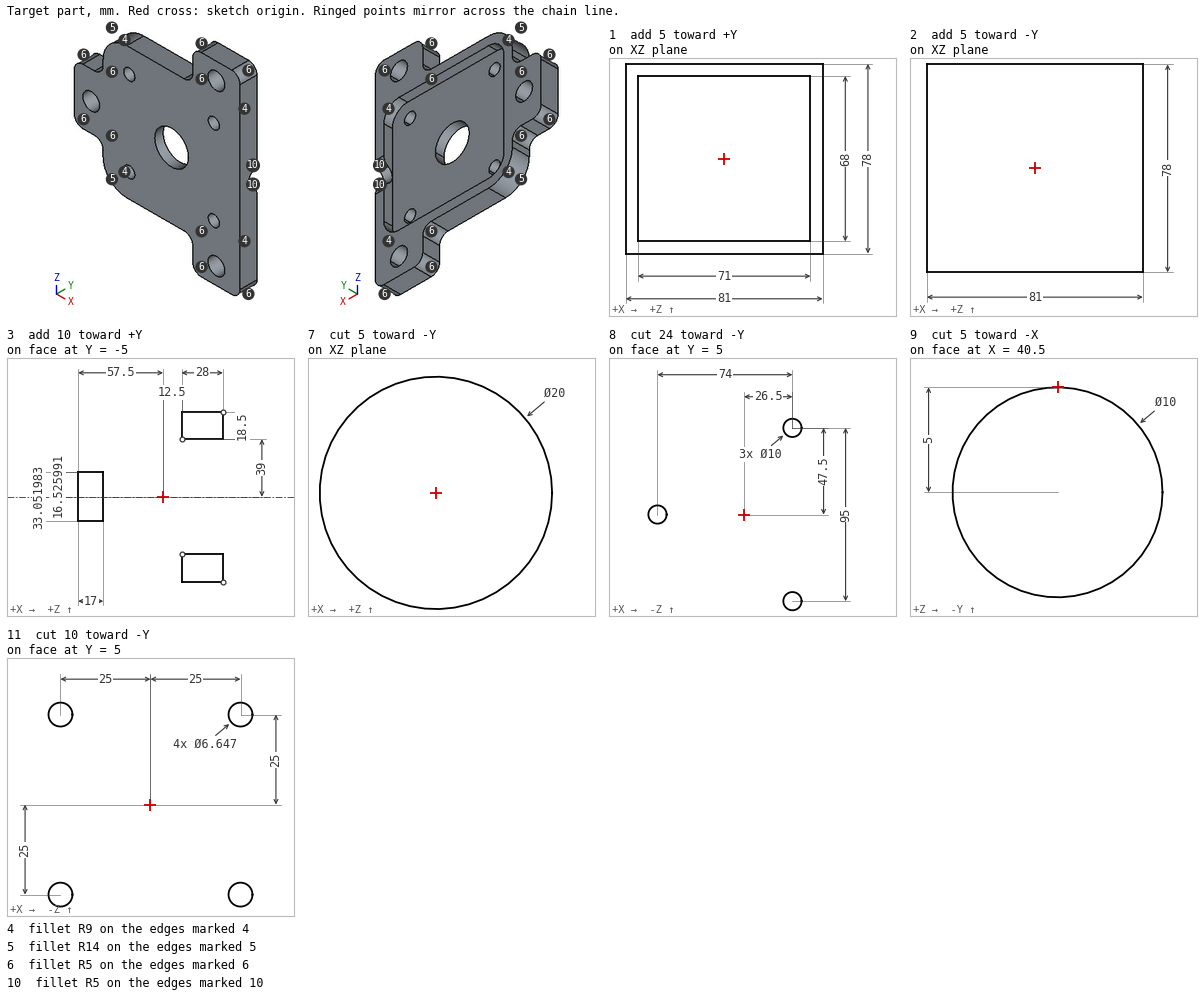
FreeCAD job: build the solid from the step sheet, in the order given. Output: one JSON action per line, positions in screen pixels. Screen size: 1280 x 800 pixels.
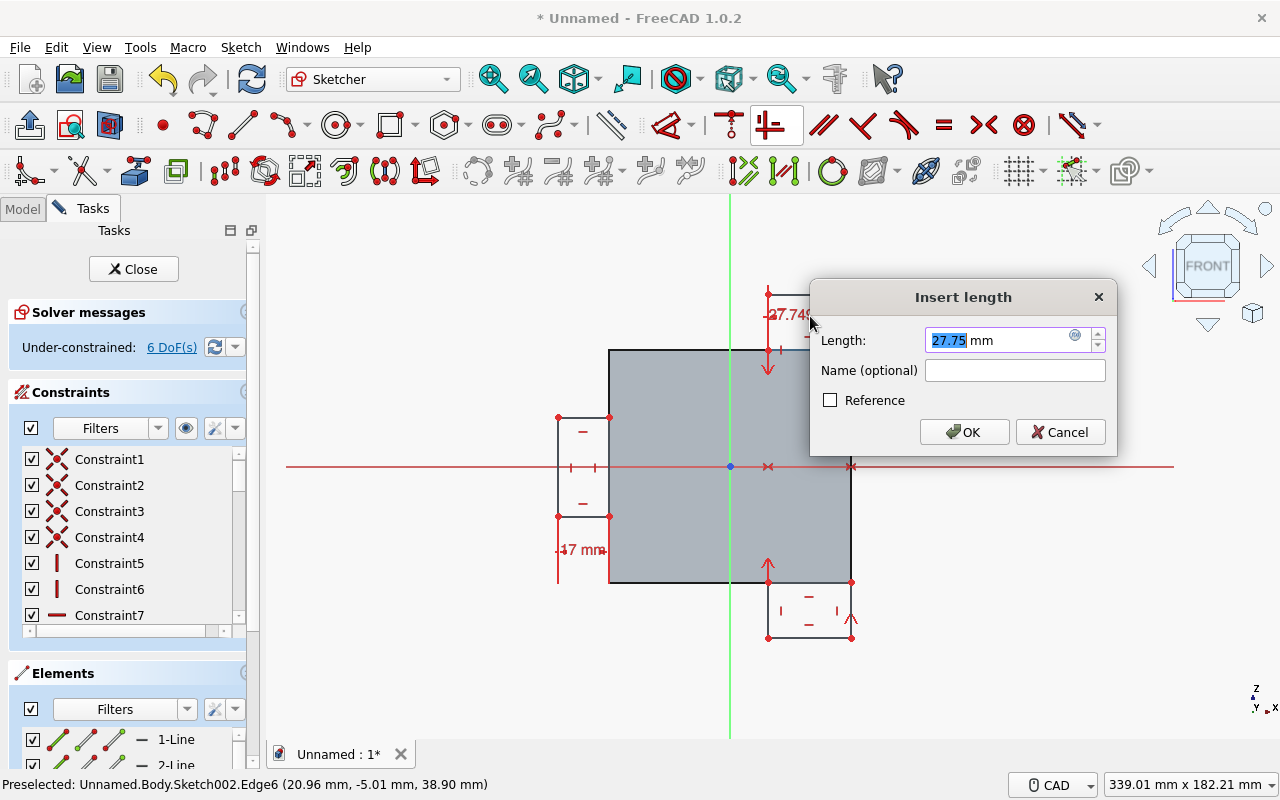
{"action": "type", "text": "28"}
{"action": "key", "text": "Return"}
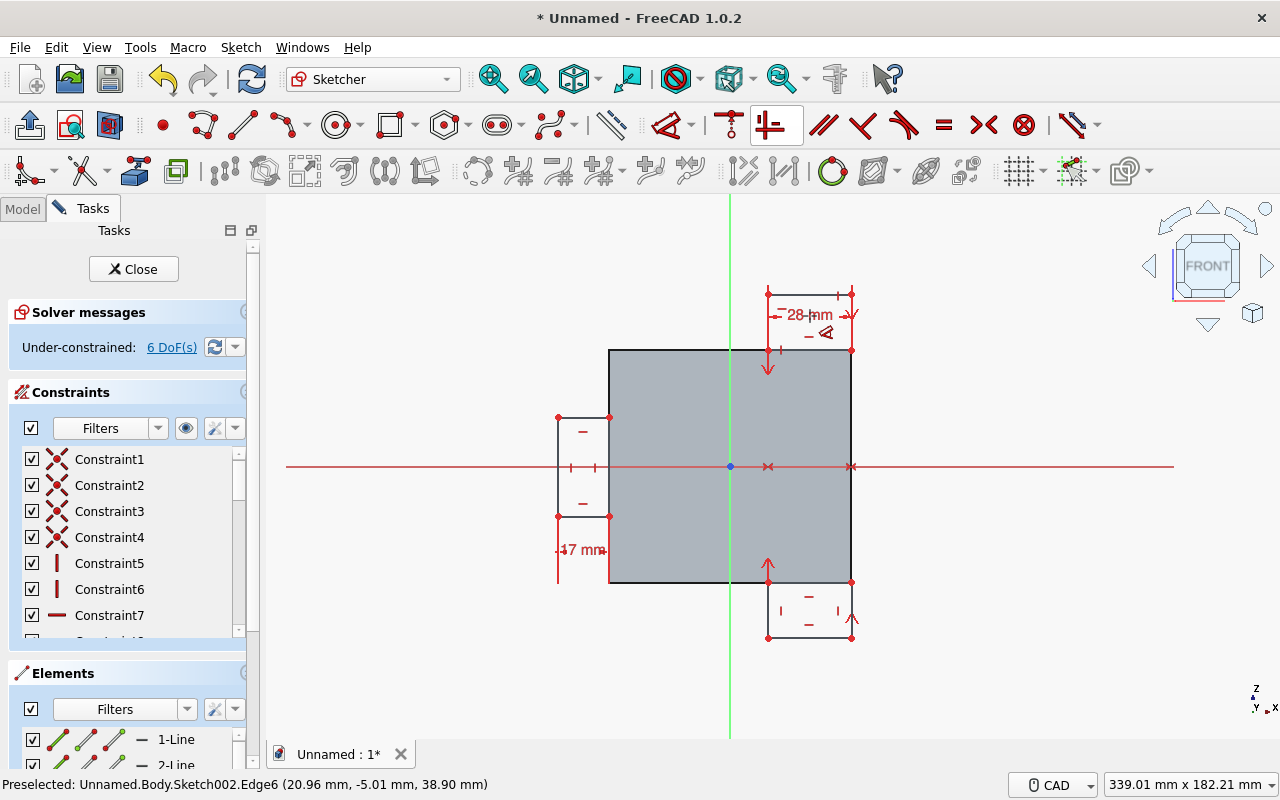
{"action": "left_click", "coordinate": [768, 350]}
{"action": "left_click", "coordinate": [802, 408]}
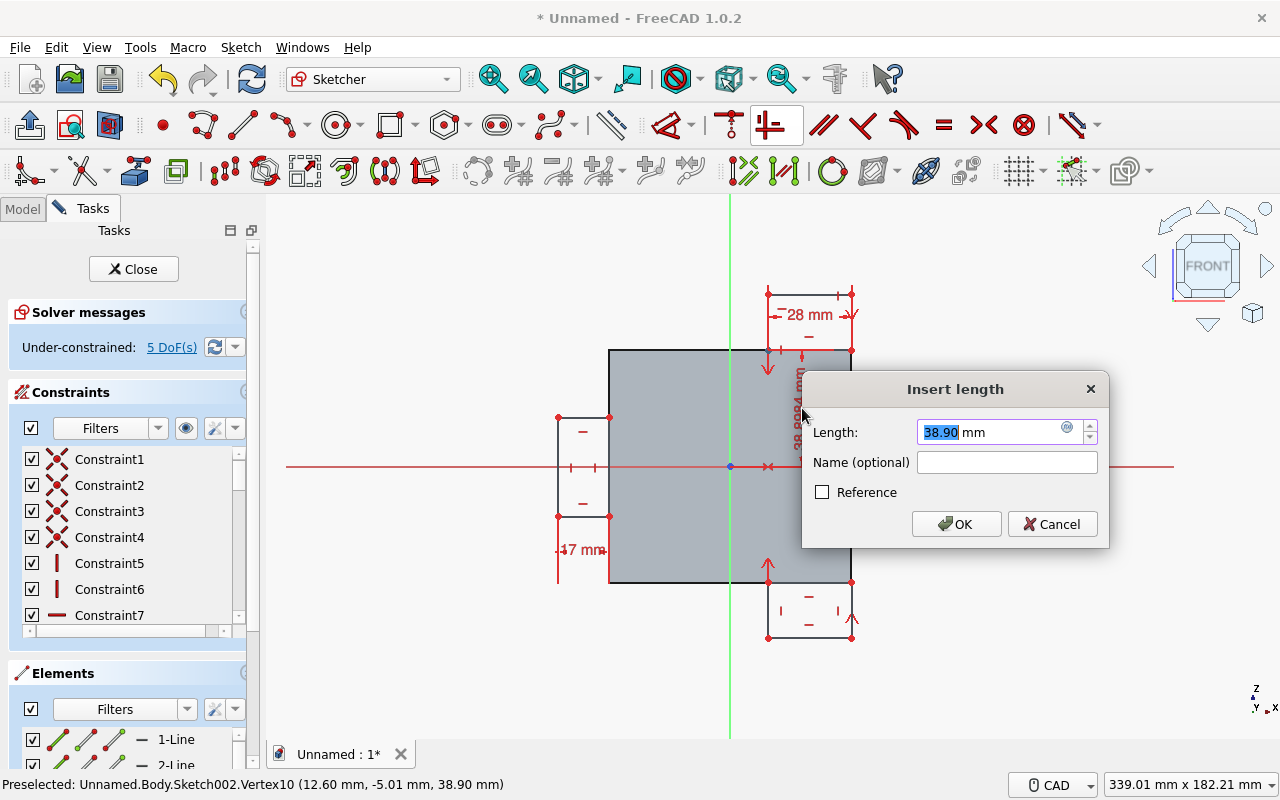
{"action": "type", "text": "39"}
{"action": "key", "text": "Return"}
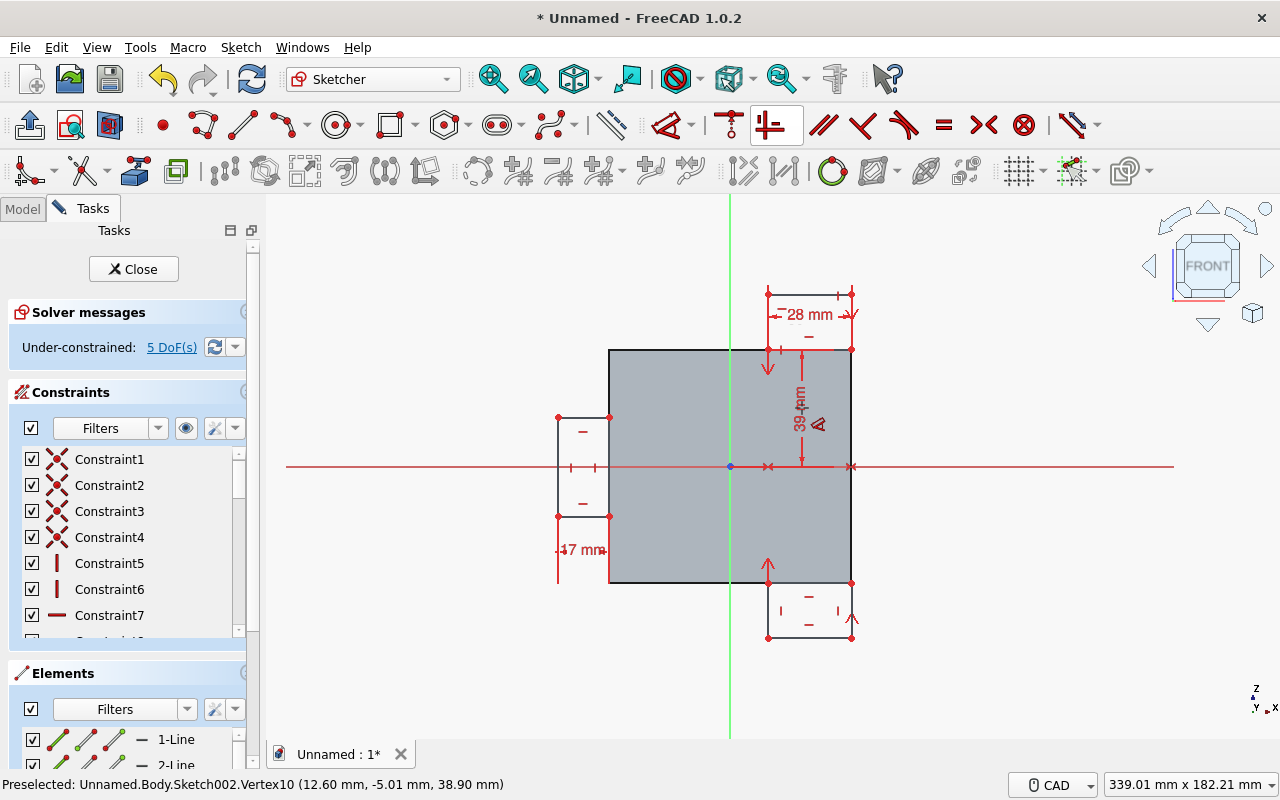
{"action": "left_click", "coordinate": [768, 311]}
{"action": "left_click", "coordinate": [710, 322]}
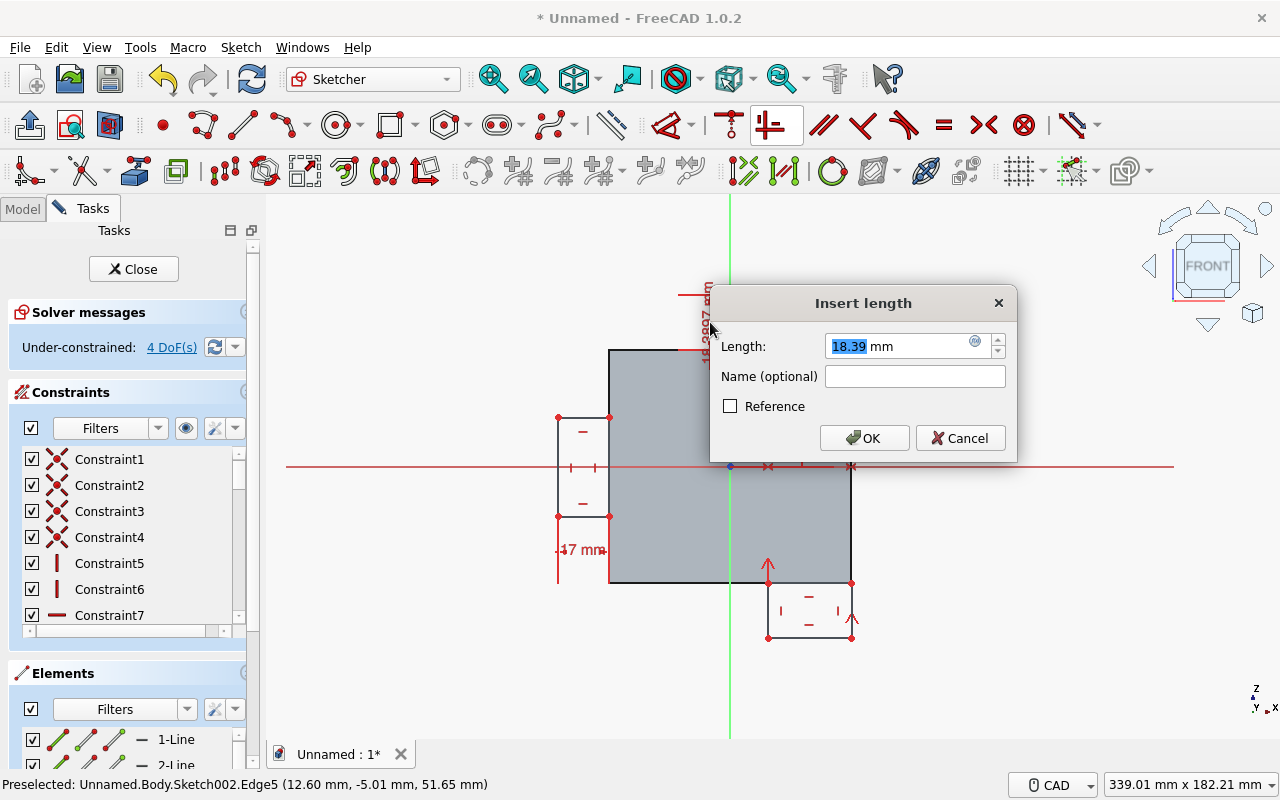
{"action": "type", "text": "18.5"}
{"action": "key", "text": "Return"}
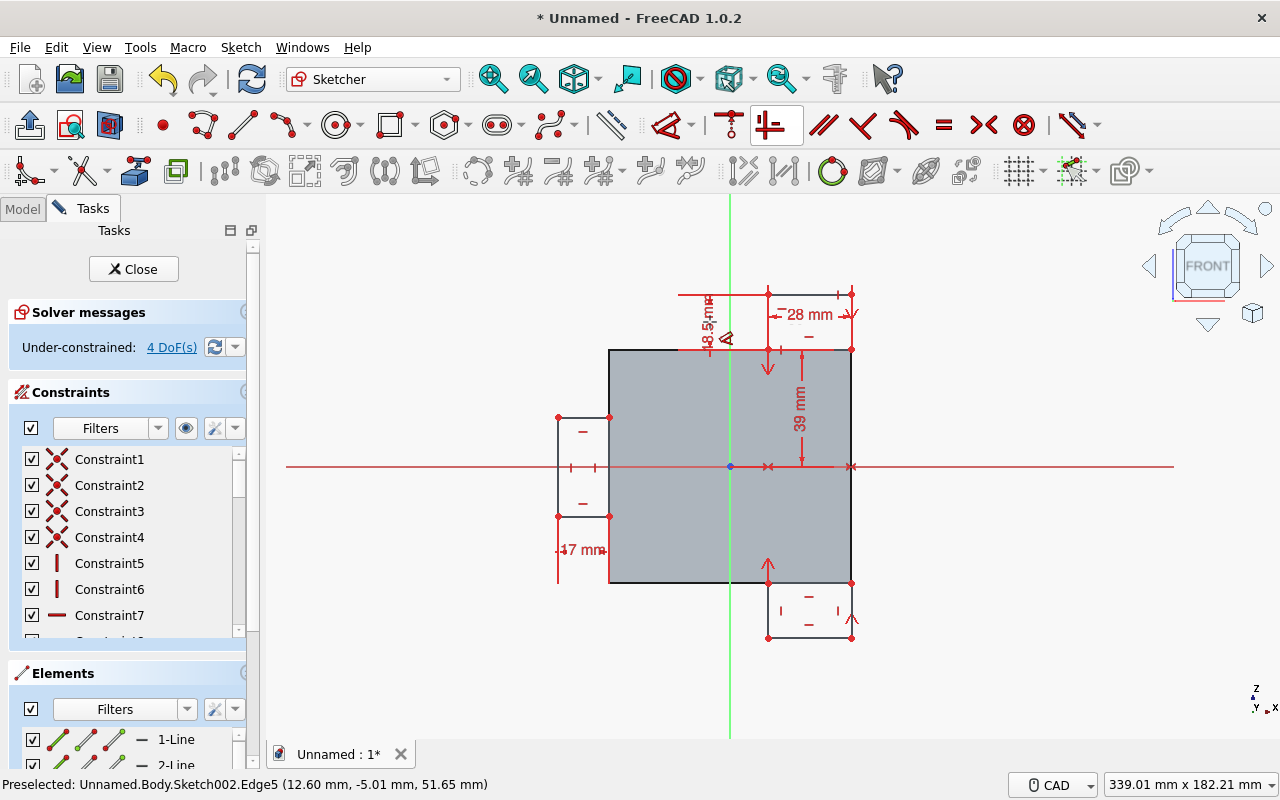
{"action": "left_click", "coordinate": [558, 418]}
{"action": "left_click", "coordinate": [644, 384]}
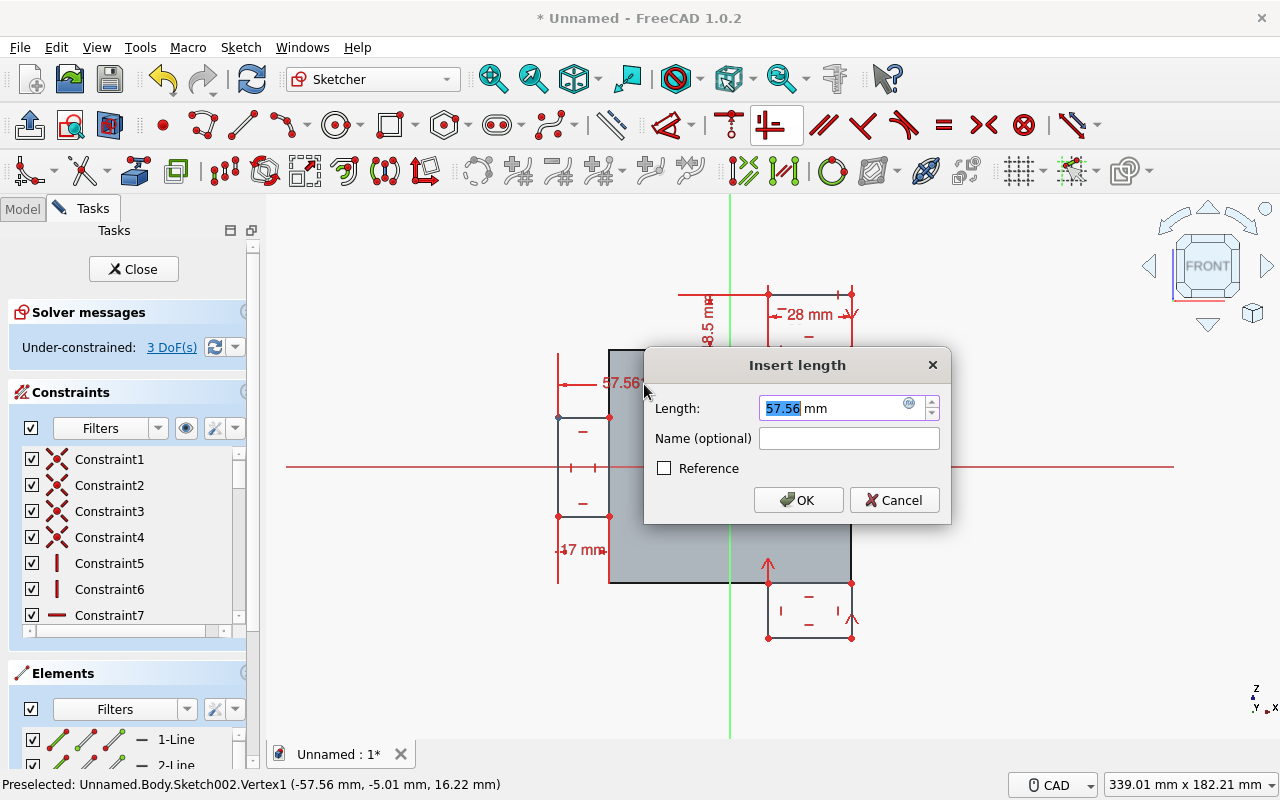
{"action": "type", "text": "57.5"}
{"action": "key", "text": "Return"}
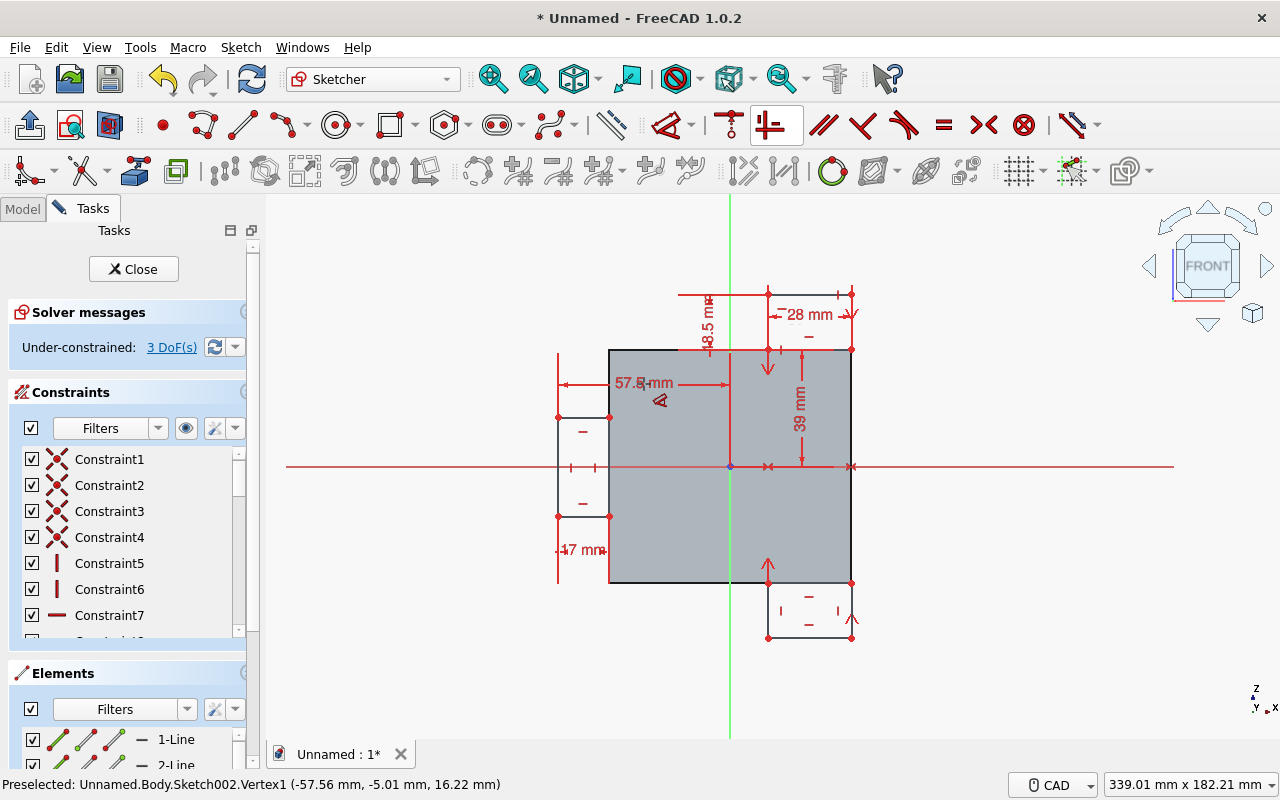
{"action": "left_click", "coordinate": [768, 295]}
{"action": "left_click", "coordinate": [749, 261]}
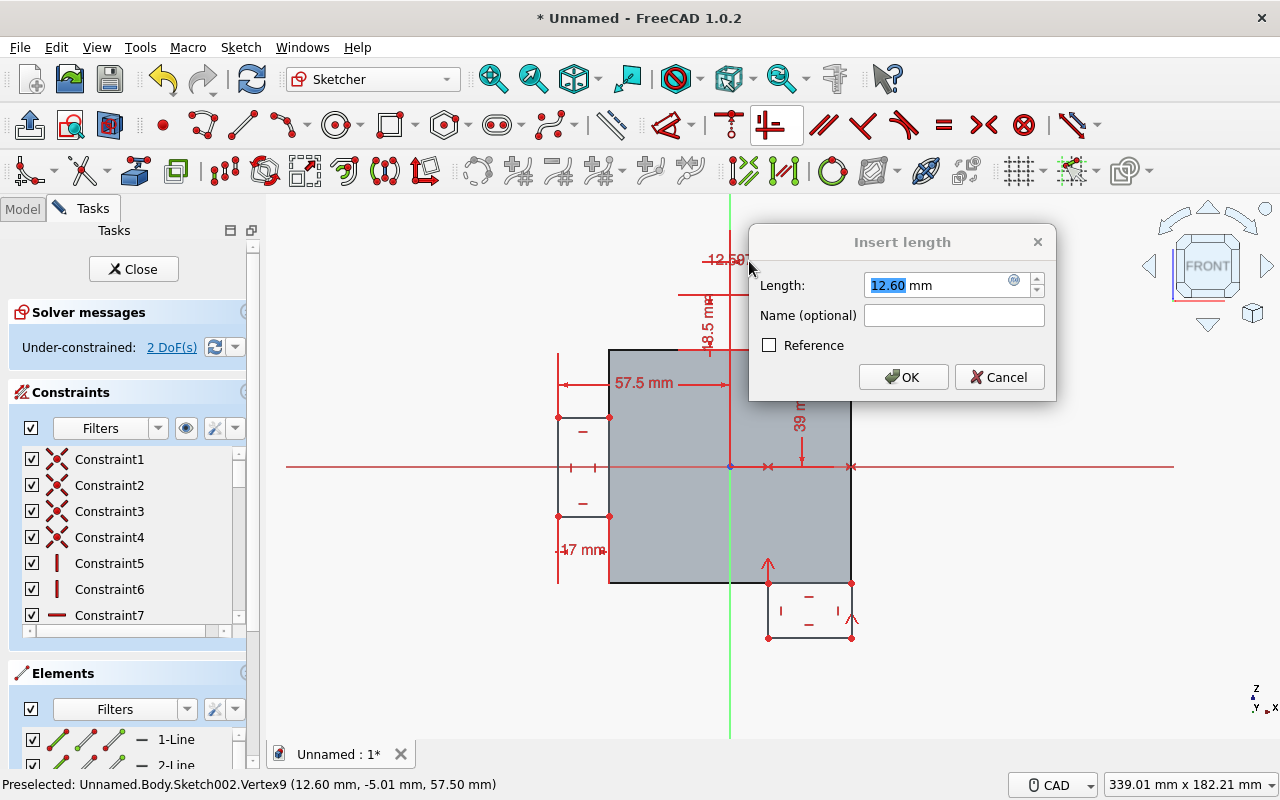
{"action": "type", "text": "12.5"}
{"action": "key", "text": "Return"}